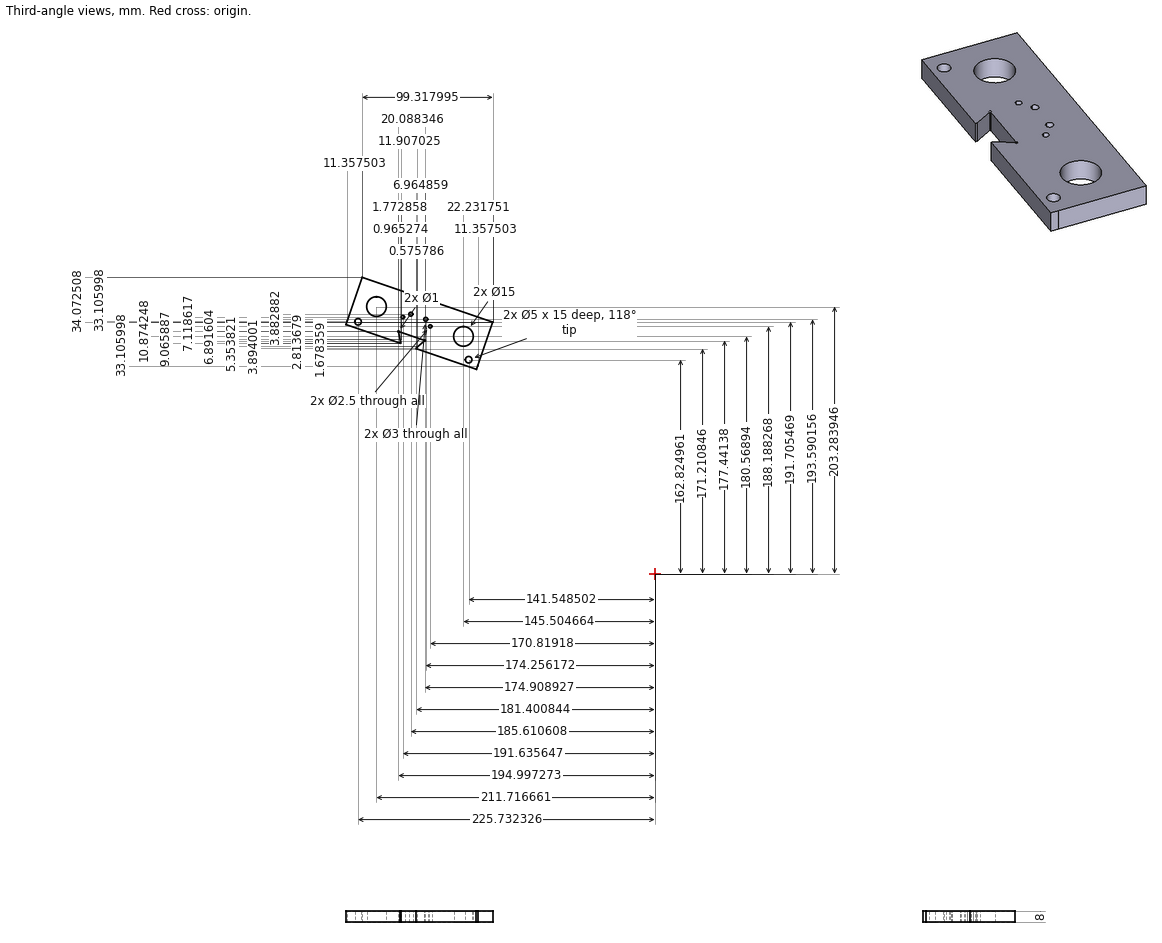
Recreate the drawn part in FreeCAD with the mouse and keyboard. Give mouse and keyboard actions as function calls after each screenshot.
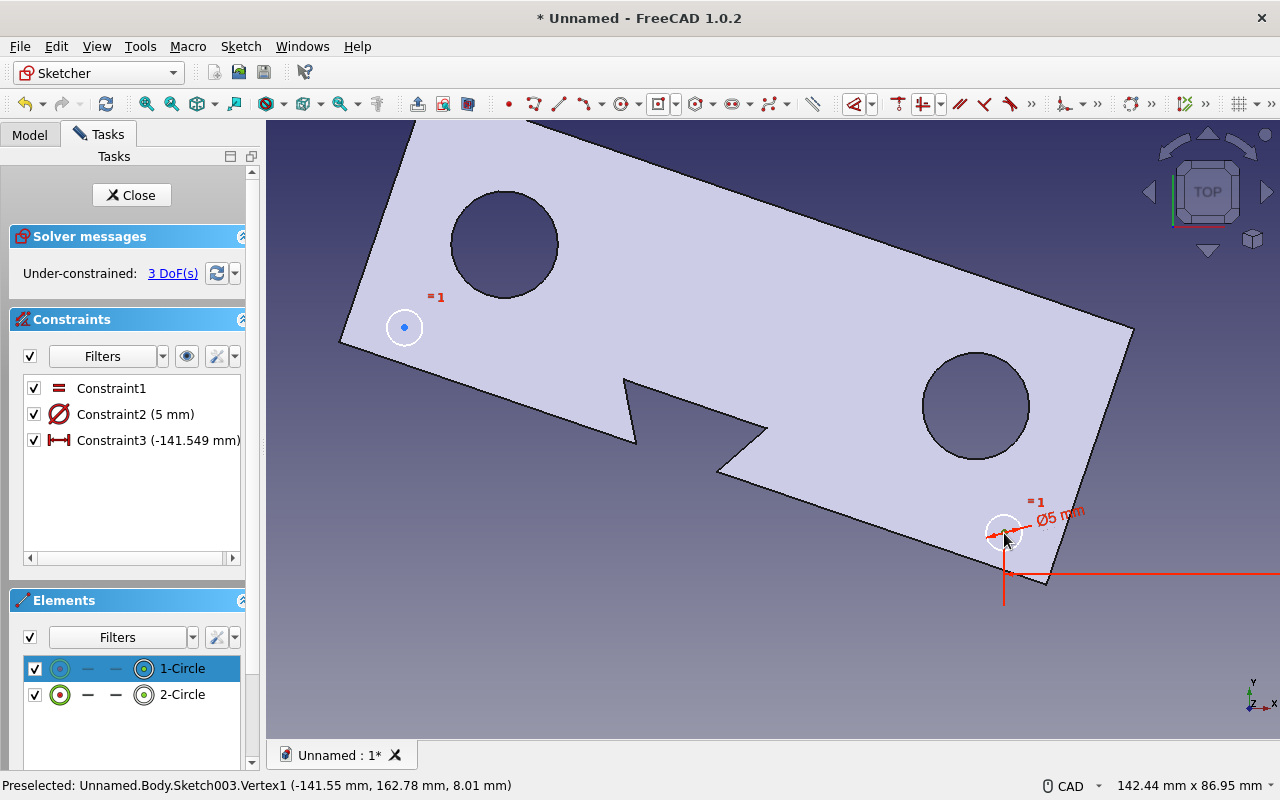
click(872, 104)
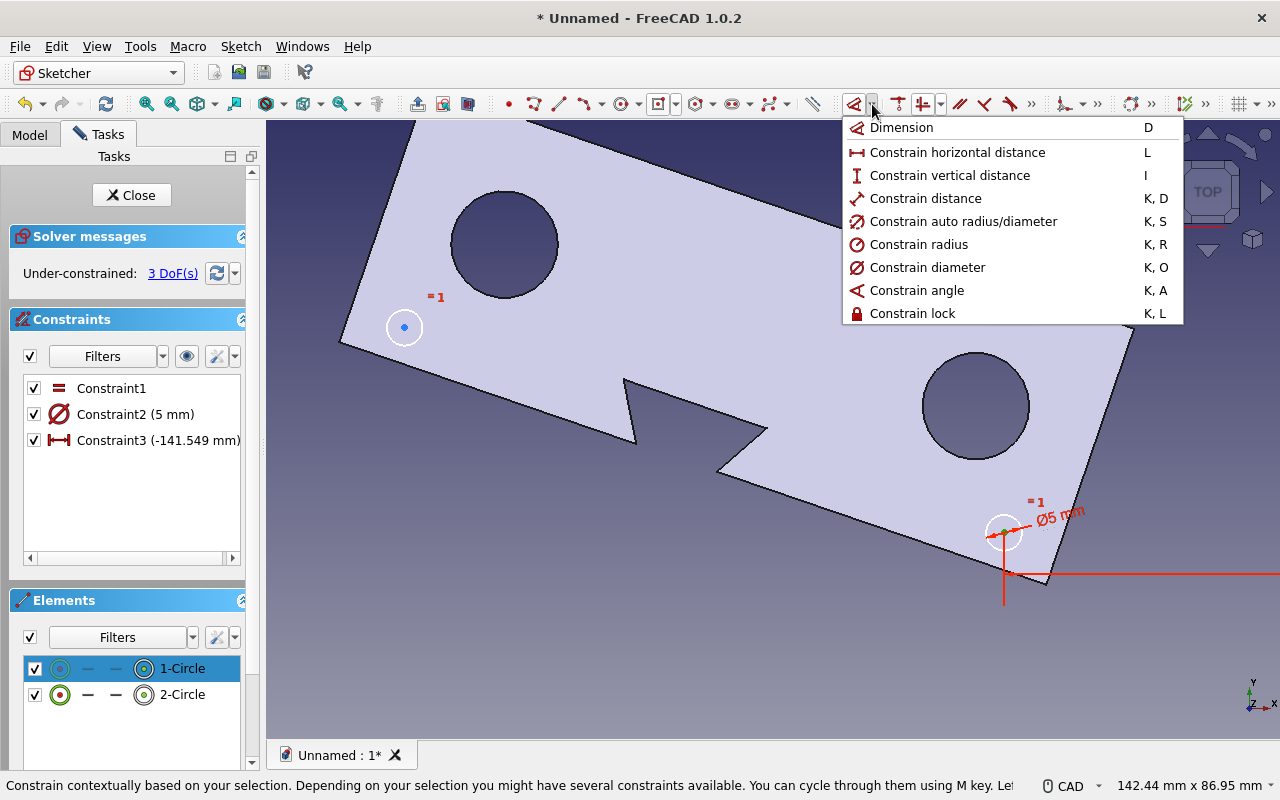
click(1013, 176)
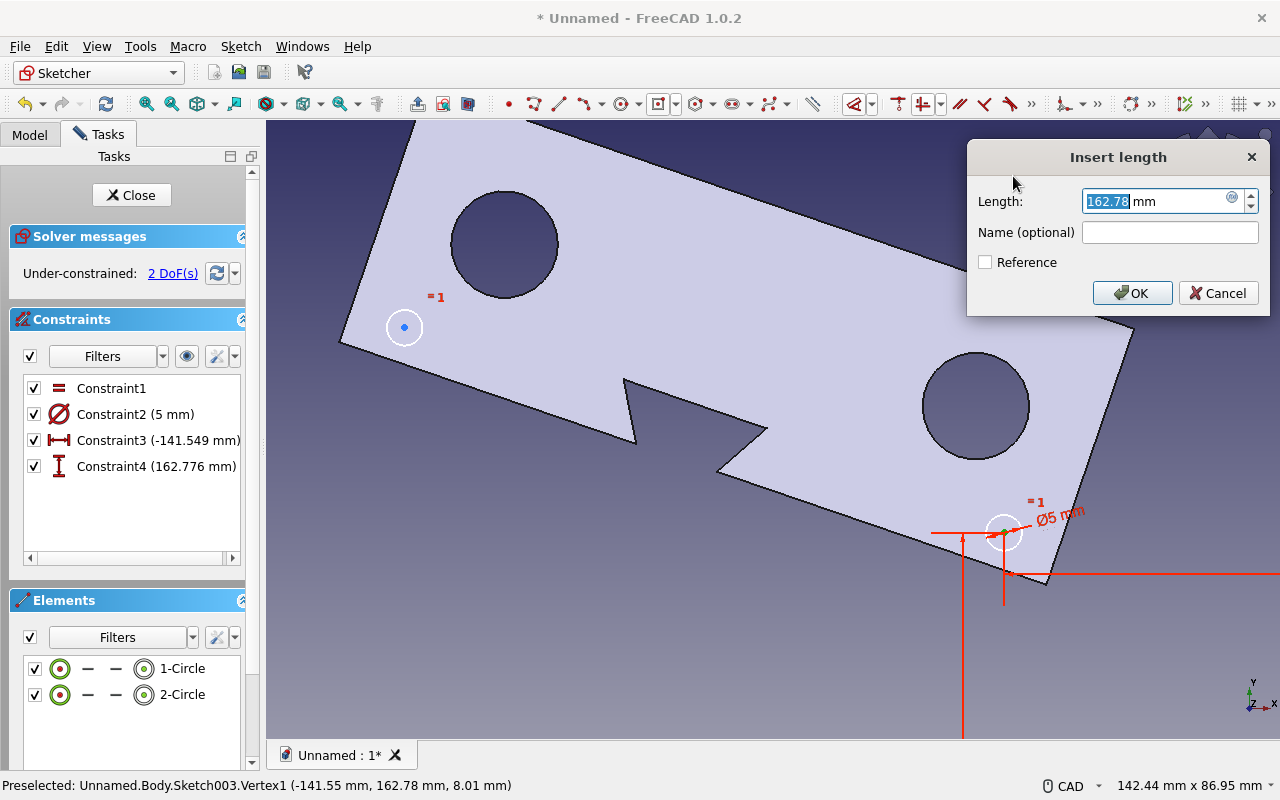
text(162.824961)
key(Return)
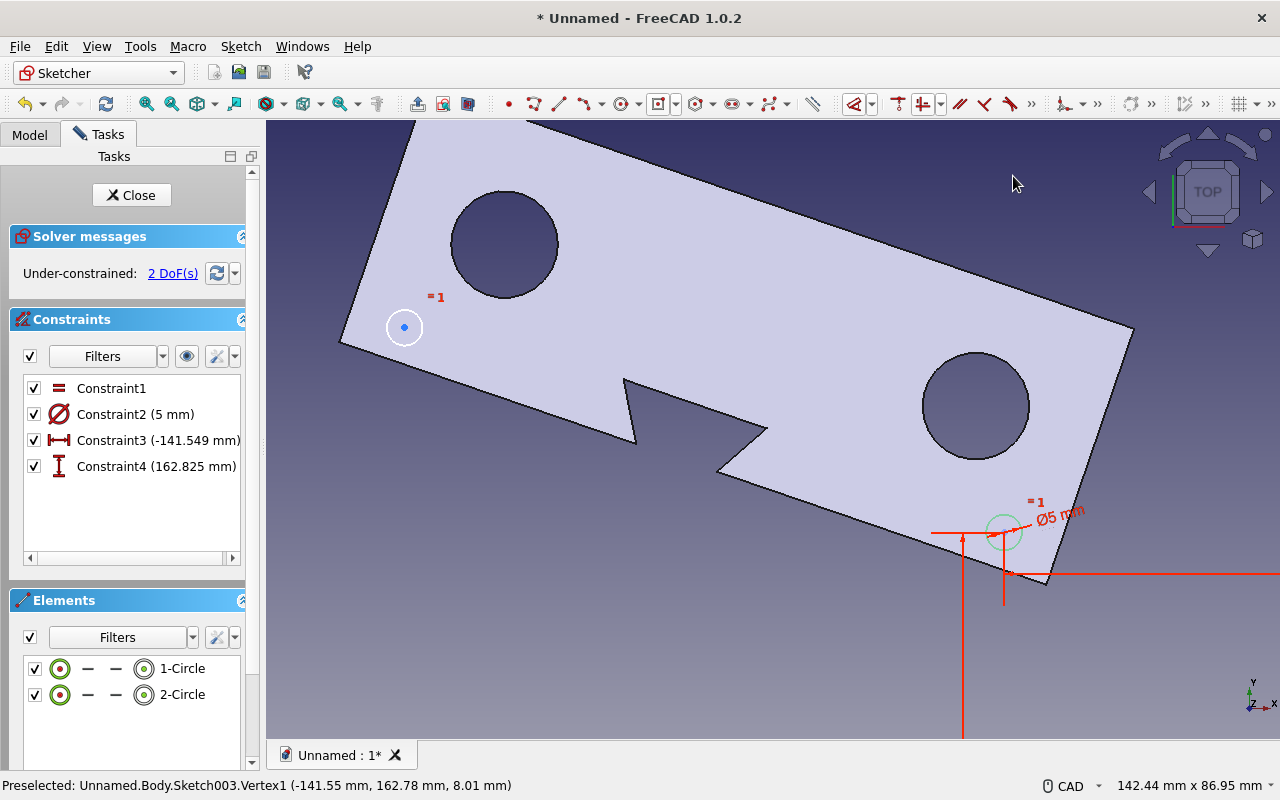
click(405, 328)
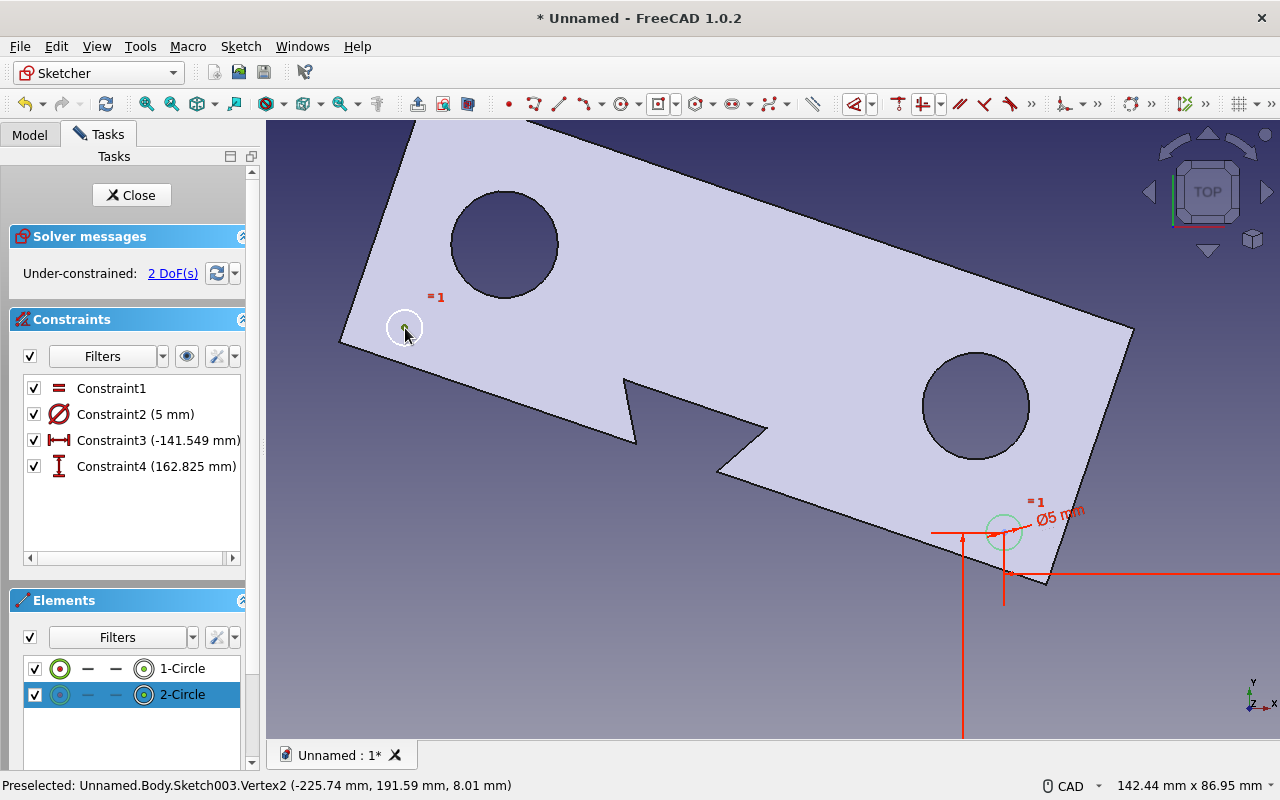
click(872, 104)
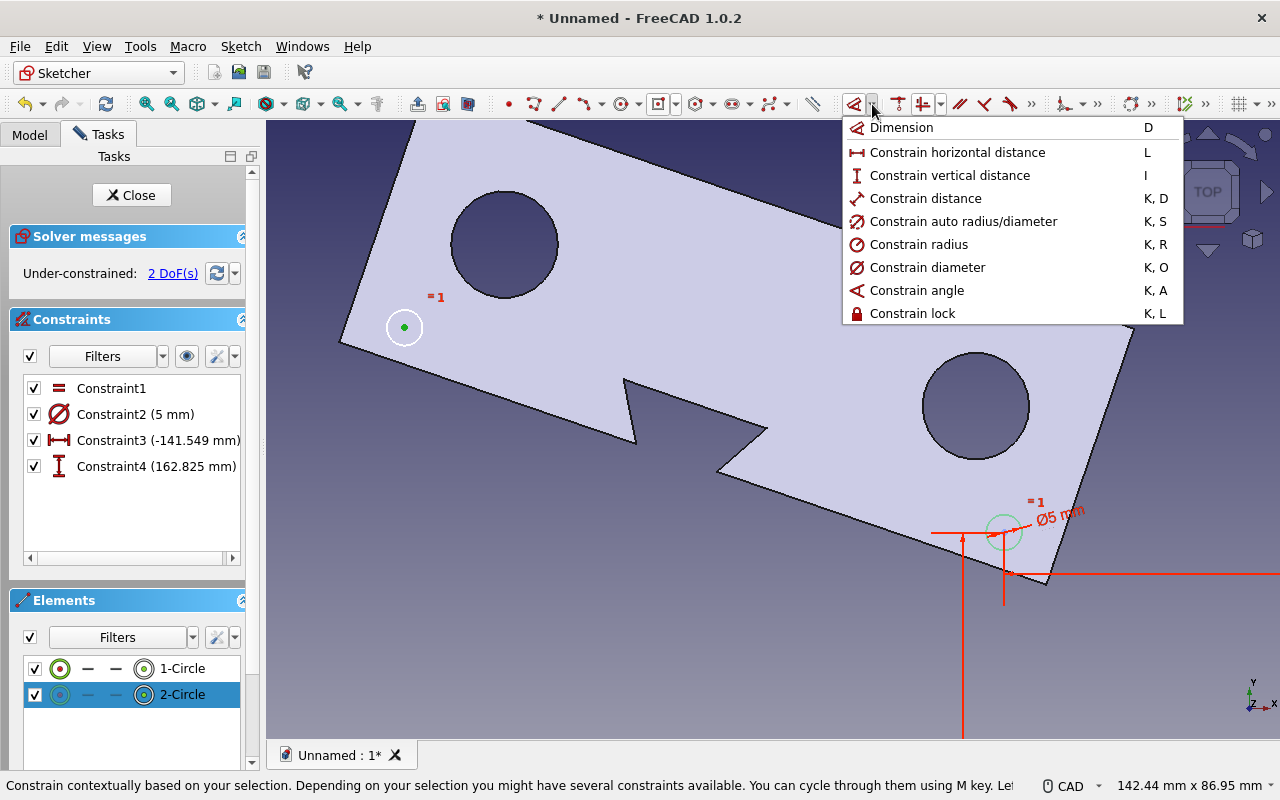
click(1013, 152)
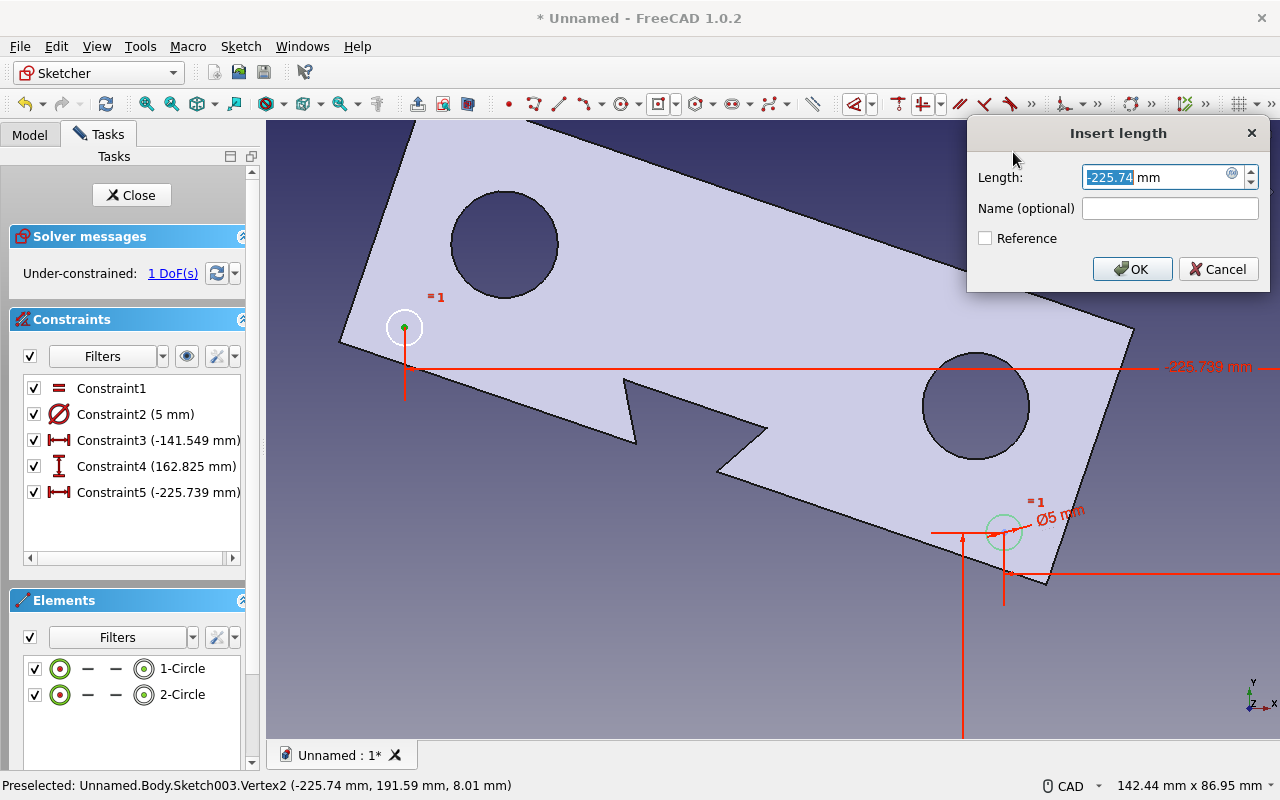
text(-225.732326)
key(Return)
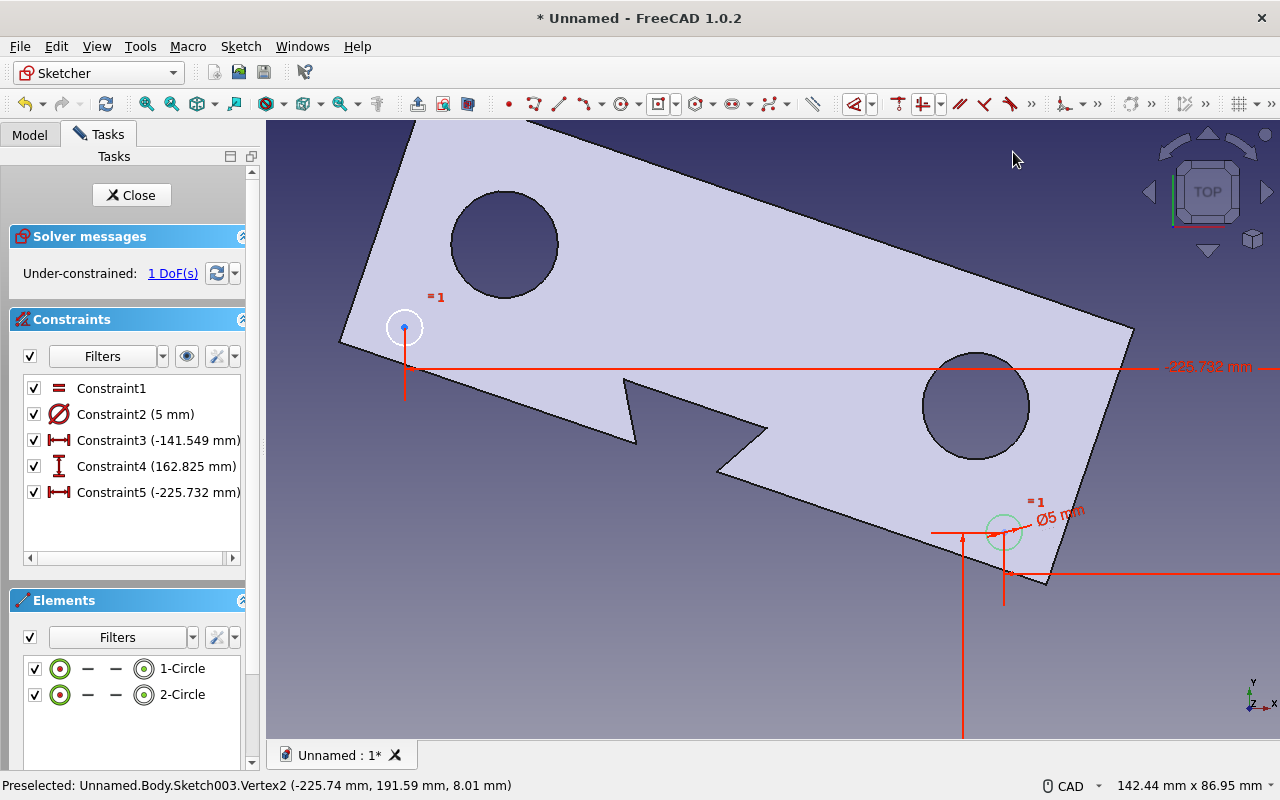
click(405, 328)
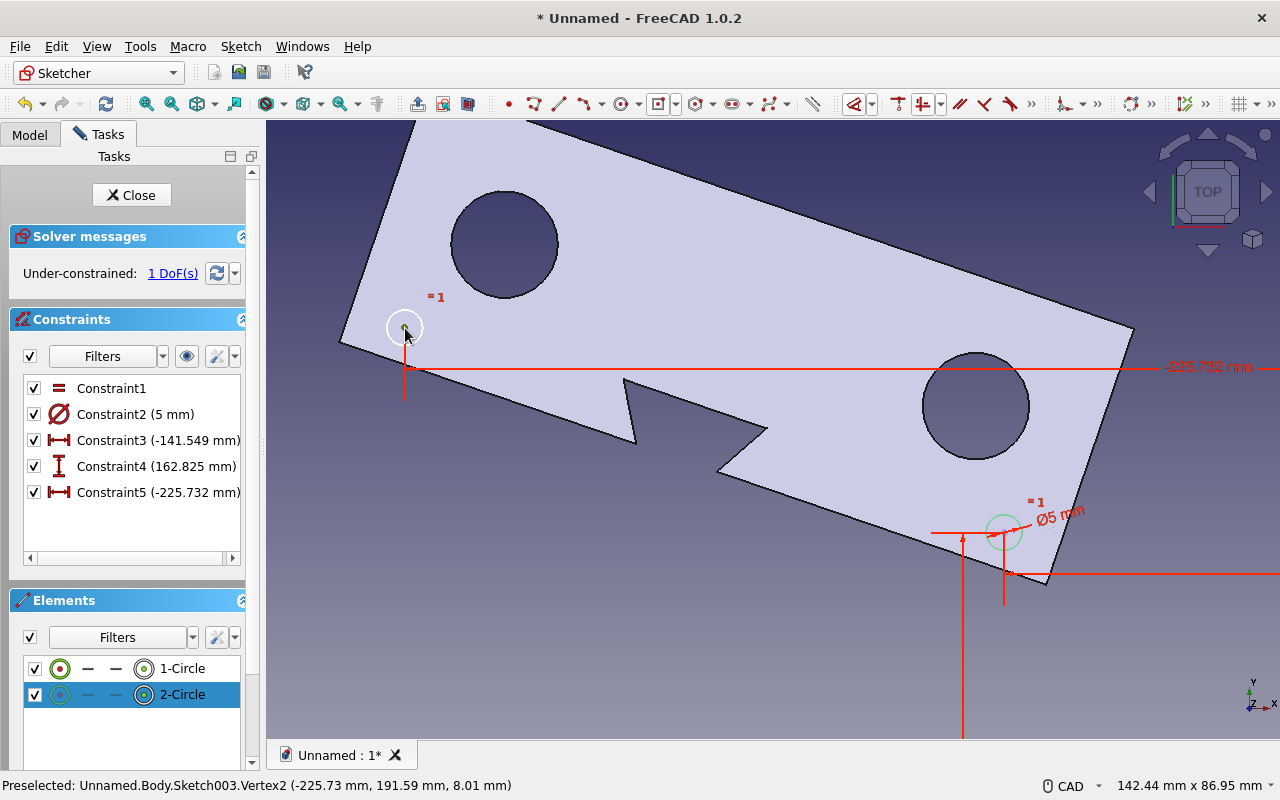
key(i)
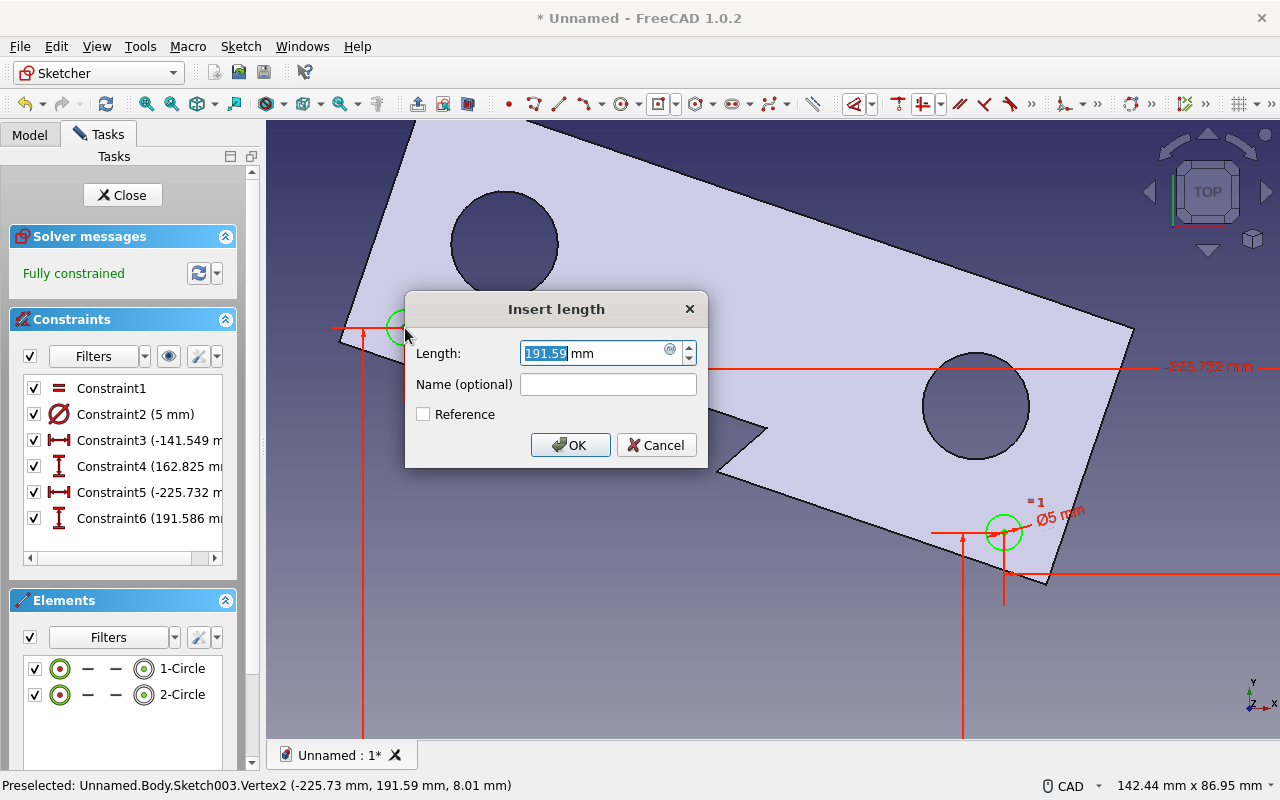
text(191.705469)
key(Return)